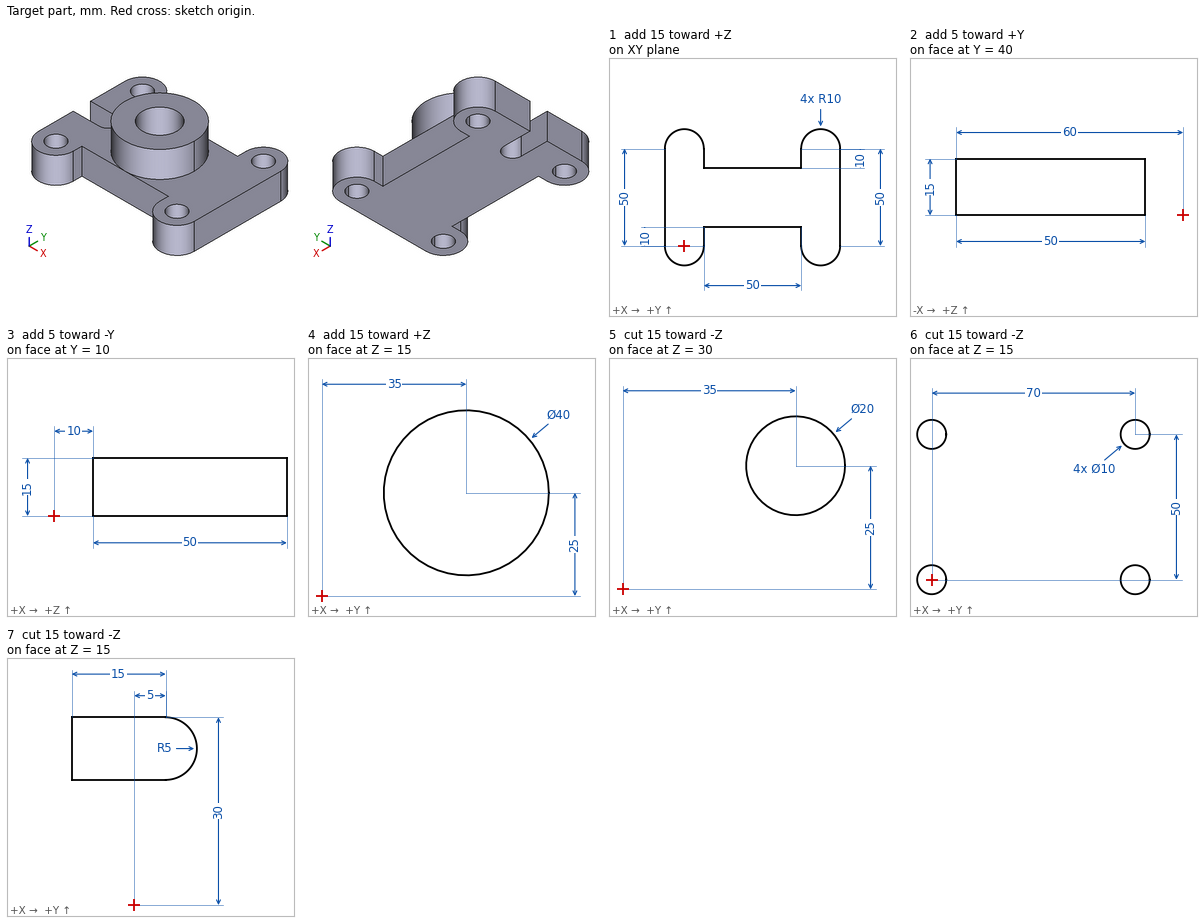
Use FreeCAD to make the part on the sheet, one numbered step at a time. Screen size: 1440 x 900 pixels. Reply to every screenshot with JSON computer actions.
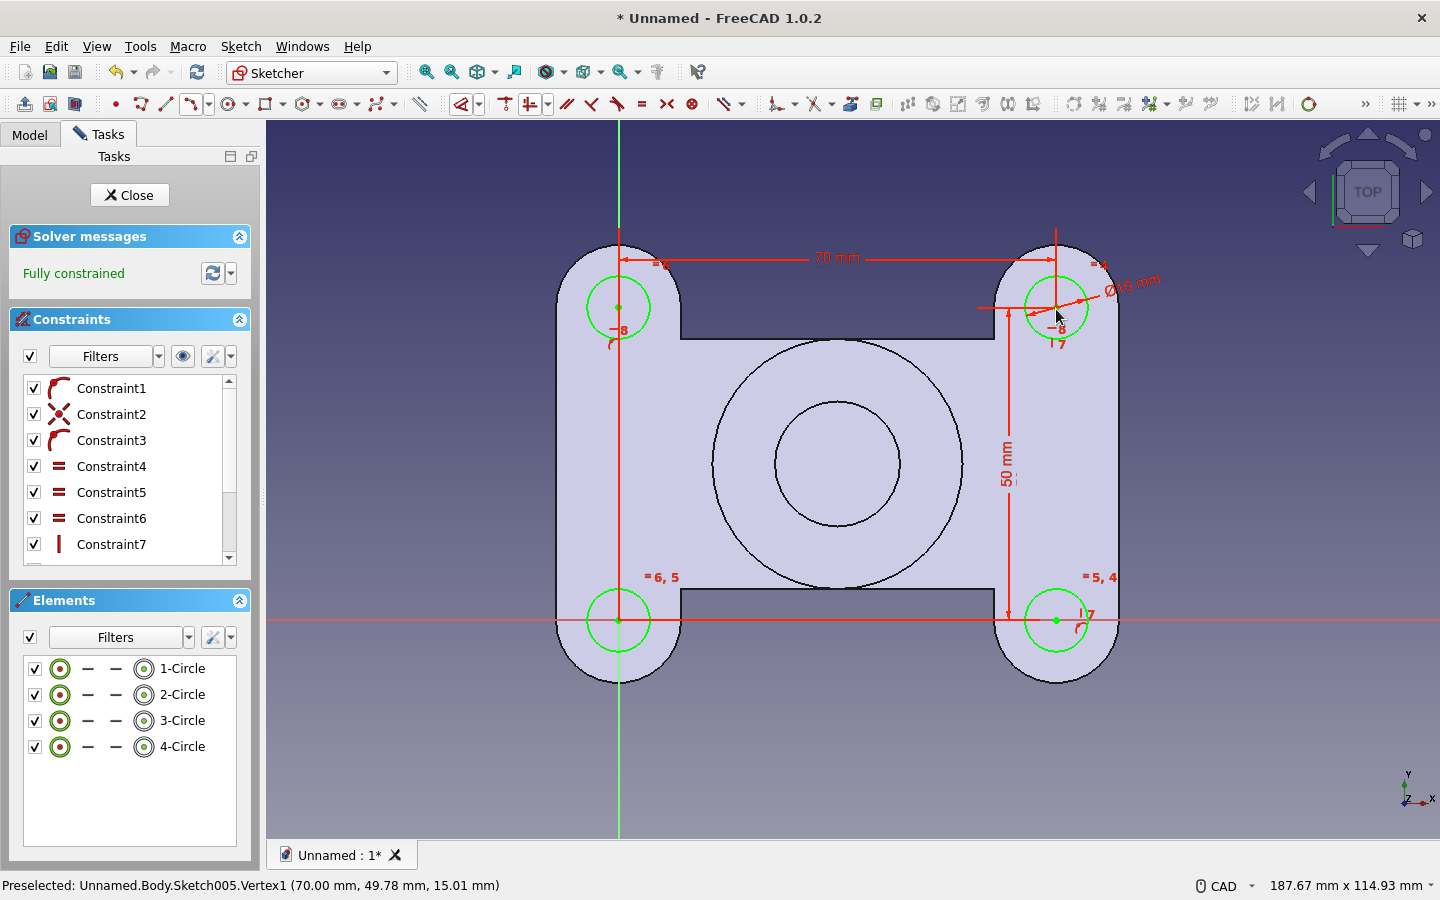
{"action": "left_click", "coordinate": [130, 195]}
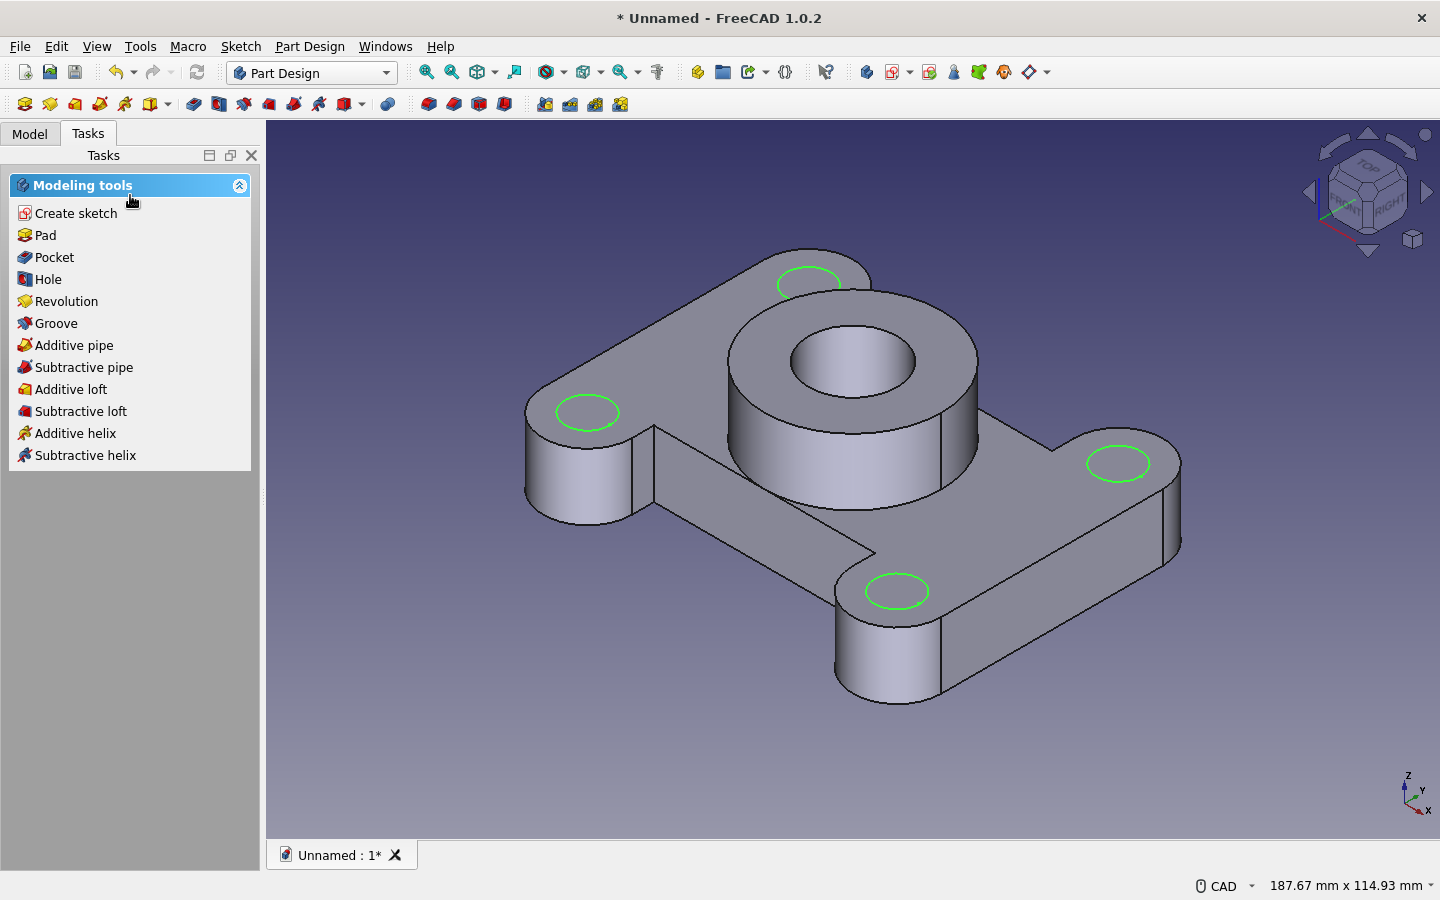
{"action": "left_click", "coordinate": [194, 104]}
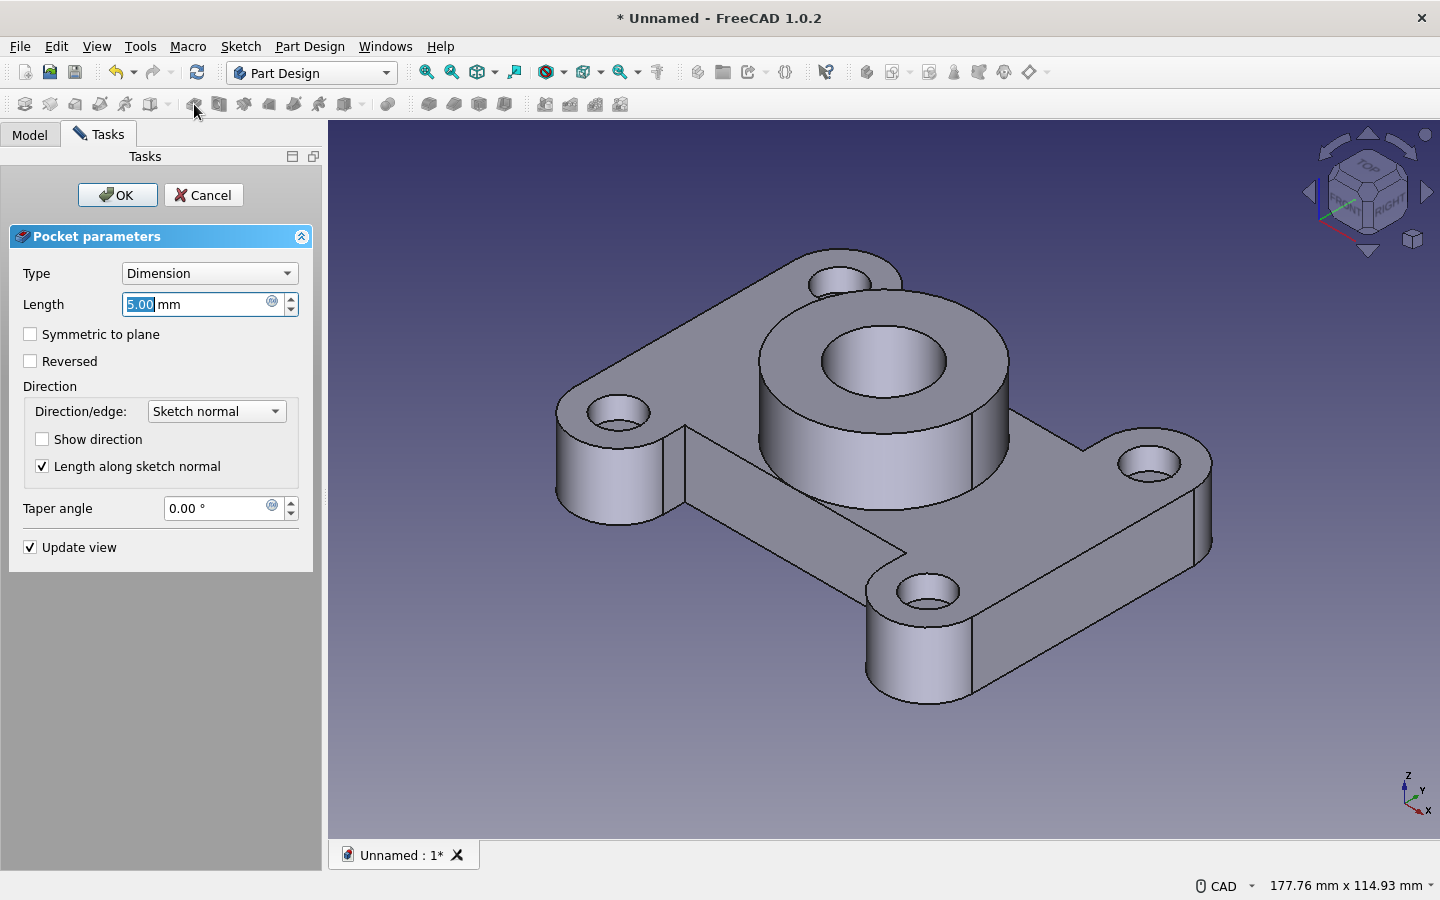
{"action": "type", "text": "15"}
{"action": "key", "text": "Tab"}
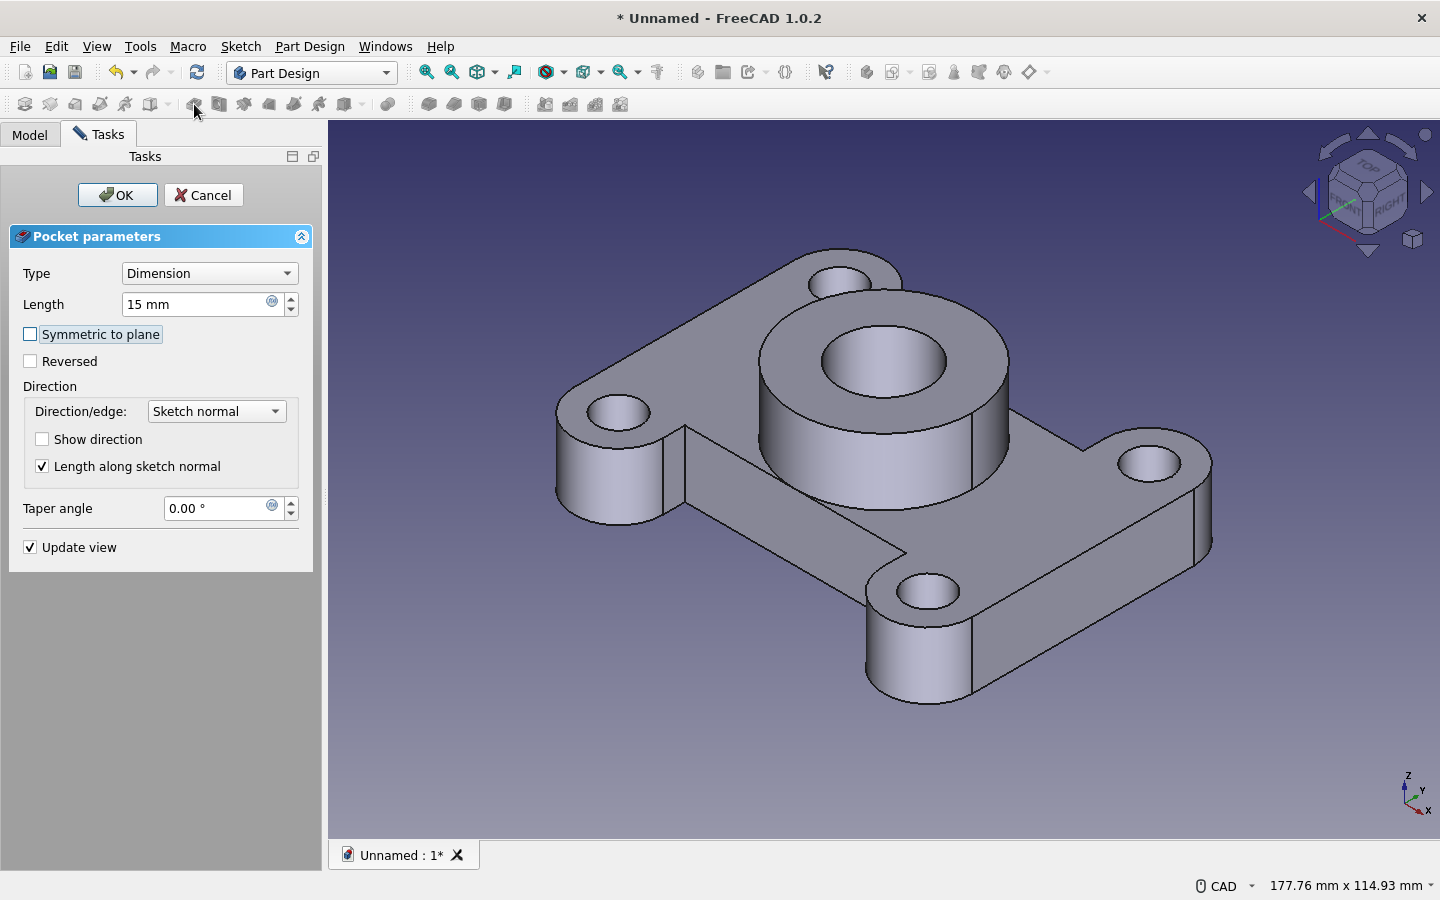
{"action": "left_click", "coordinate": [118, 195]}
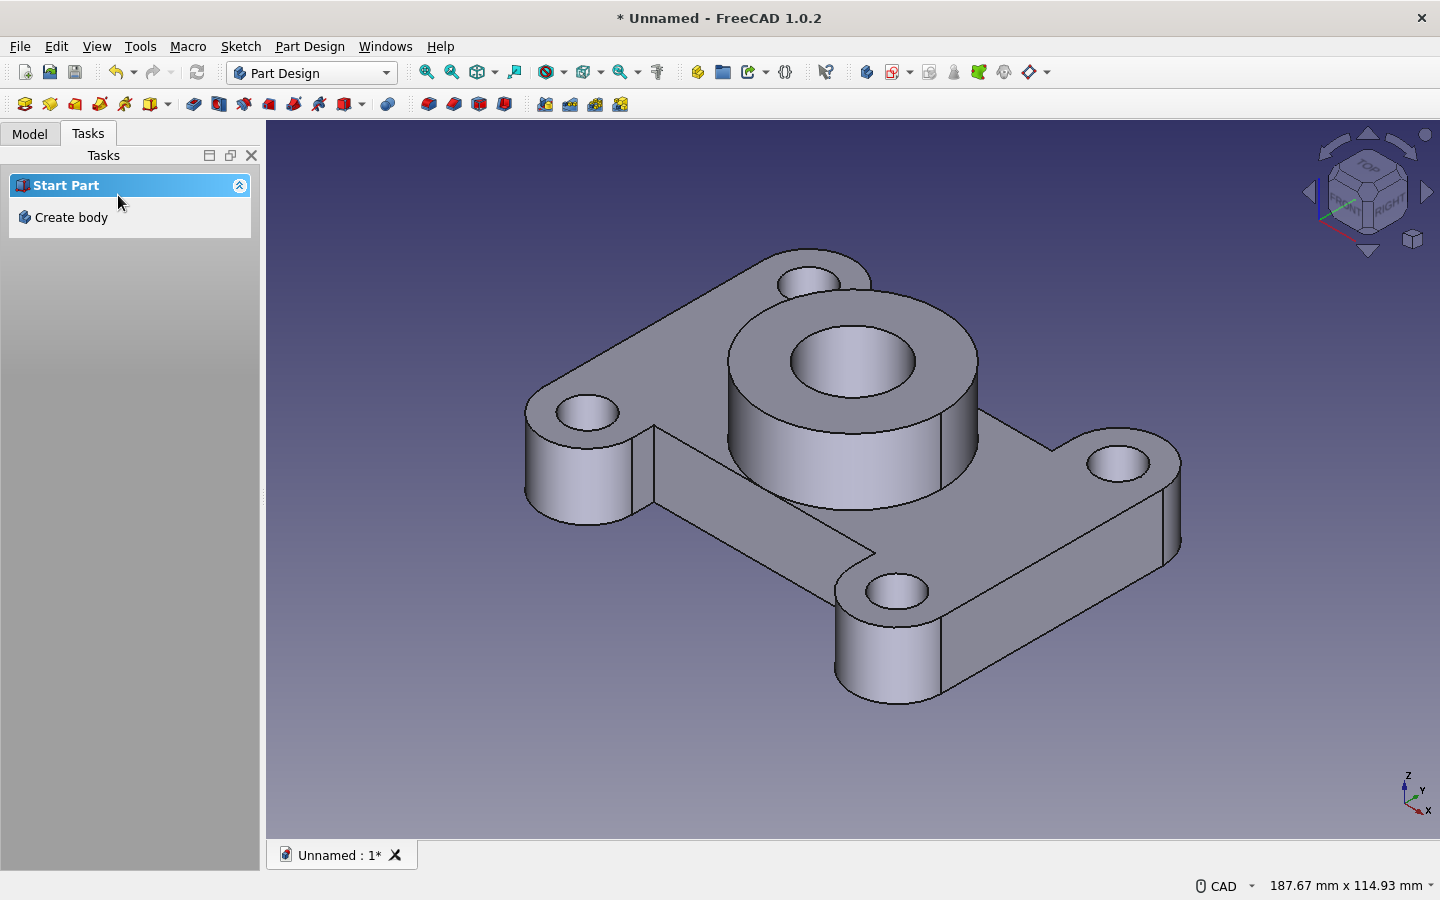
{"action": "left_click", "coordinate": [1025, 486]}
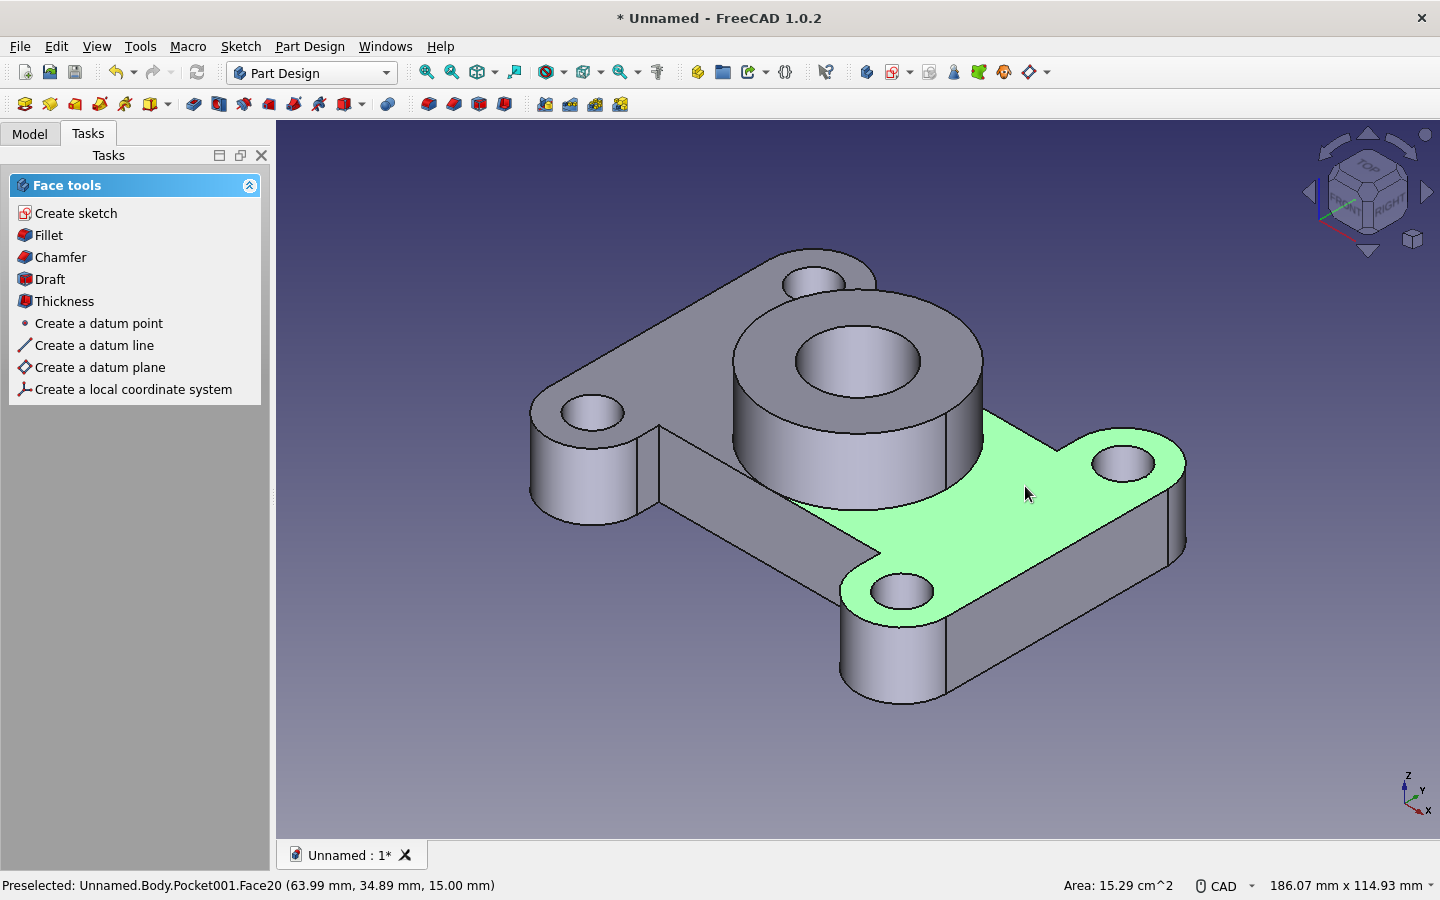
{"action": "left_click", "coordinate": [892, 72]}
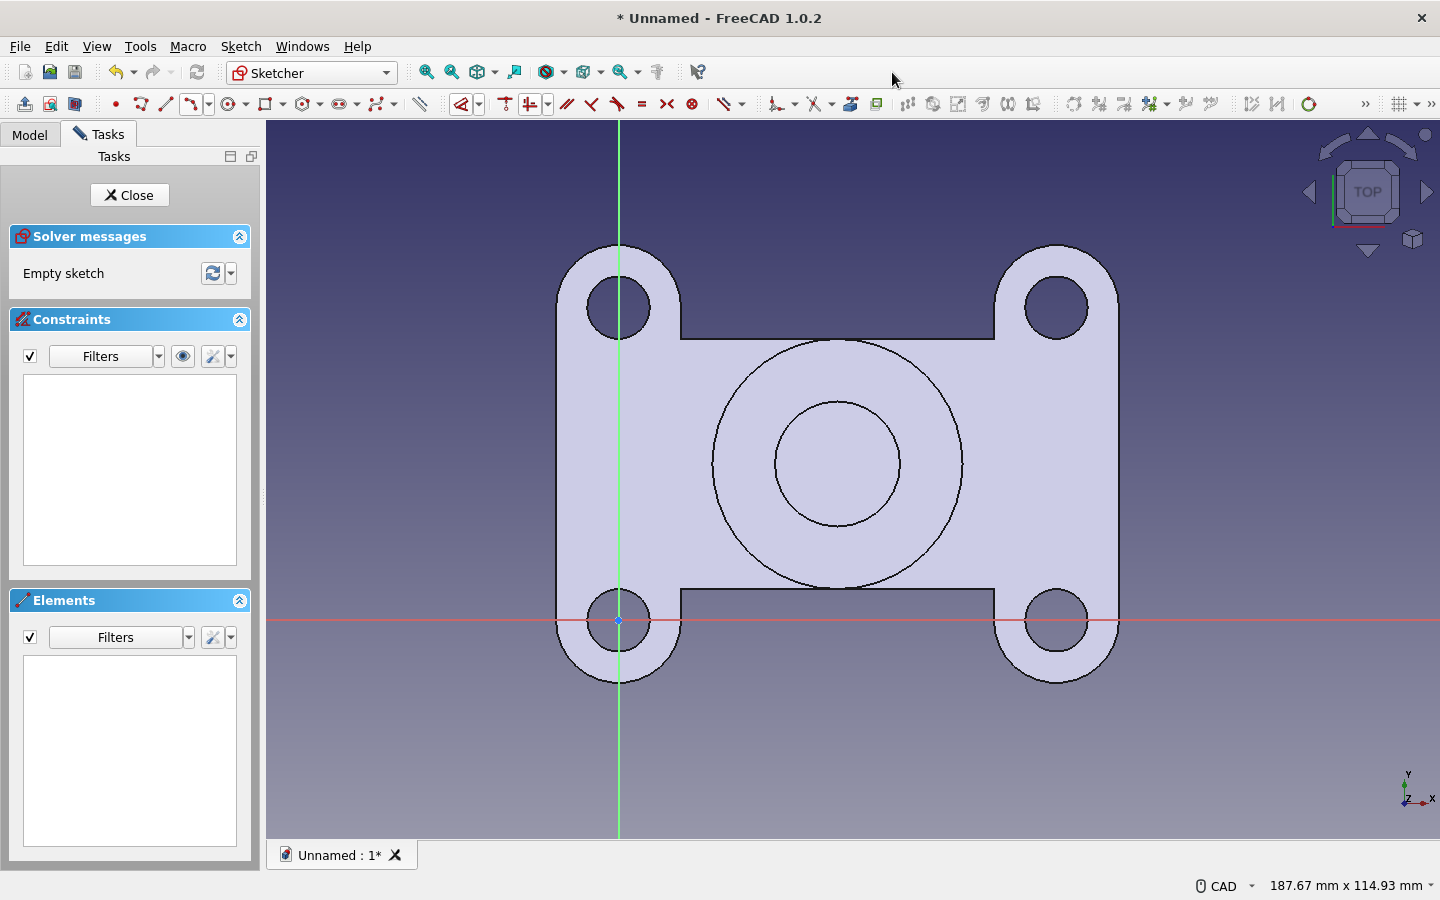
{"action": "scroll", "coordinate": [522, 554], "scroll_direction": "up", "scroll_amount": 5}